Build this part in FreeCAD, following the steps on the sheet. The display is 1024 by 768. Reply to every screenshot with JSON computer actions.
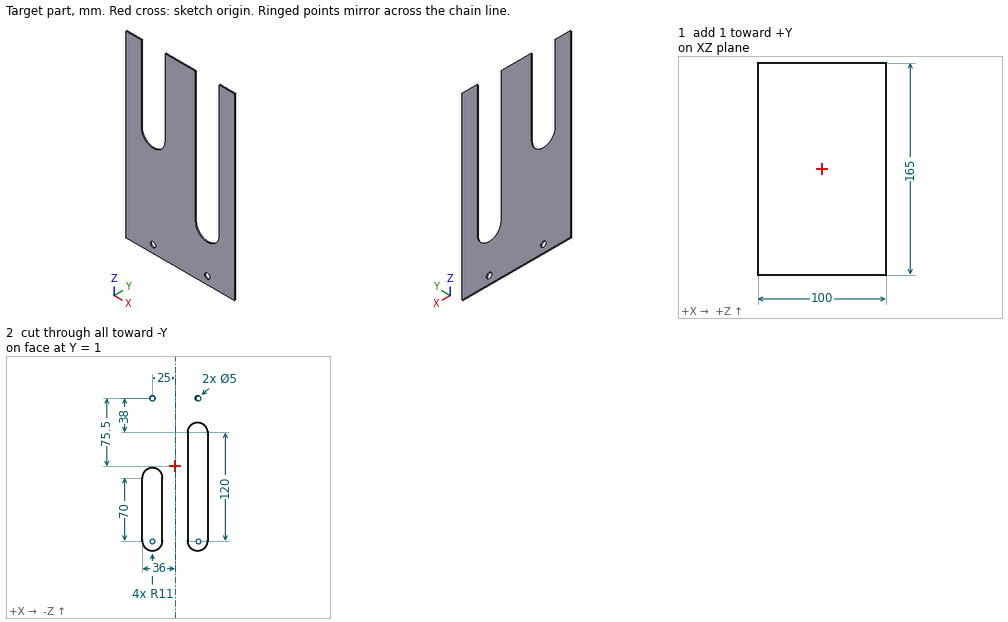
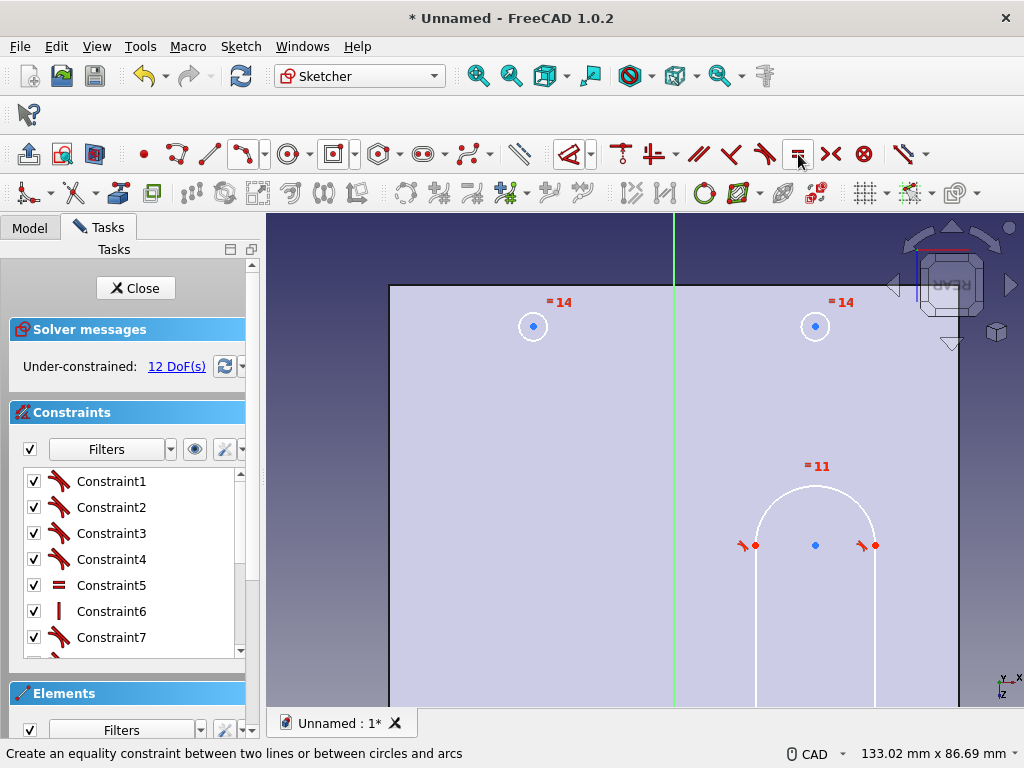
{"action": "scroll", "coordinate": [534, 314], "scroll_direction": "down", "scroll_amount": 6}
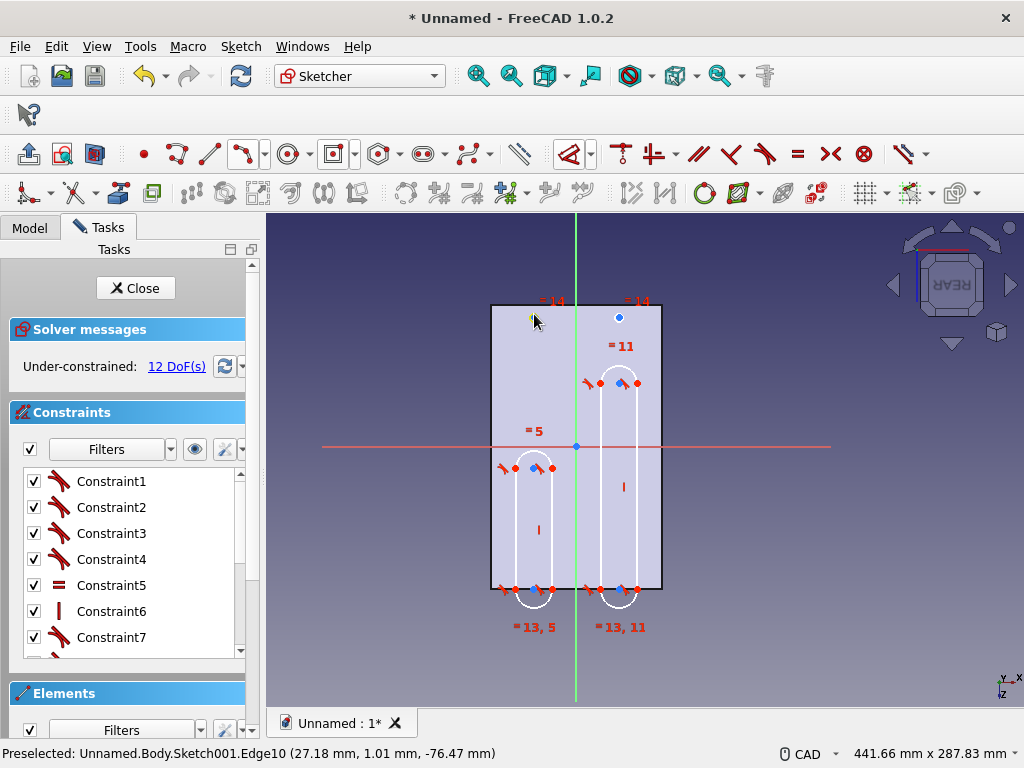
{"action": "left_click", "coordinate": [534, 590]}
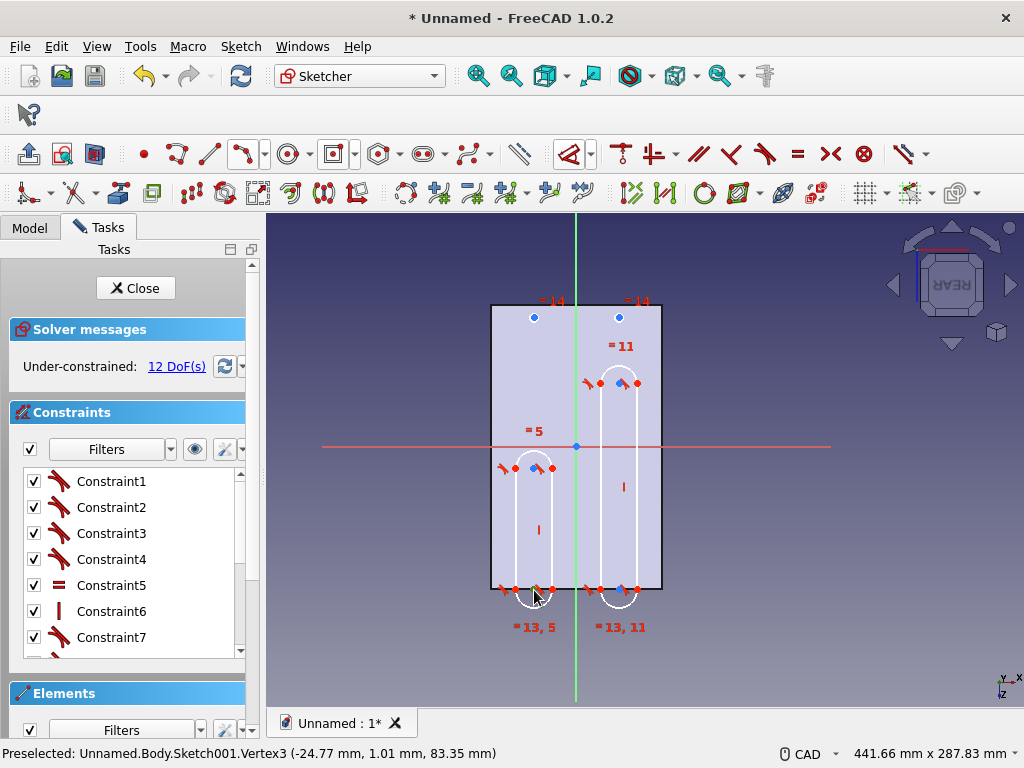
{"action": "left_click", "coordinate": [619, 590]}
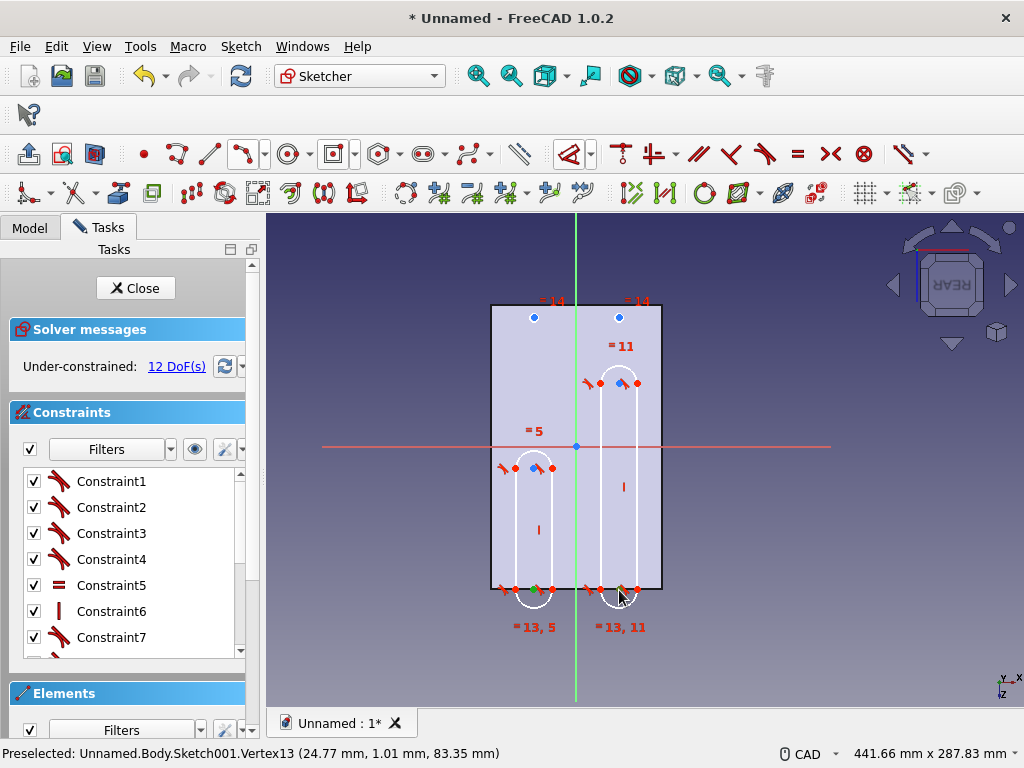
{"action": "left_click", "coordinate": [577, 648]}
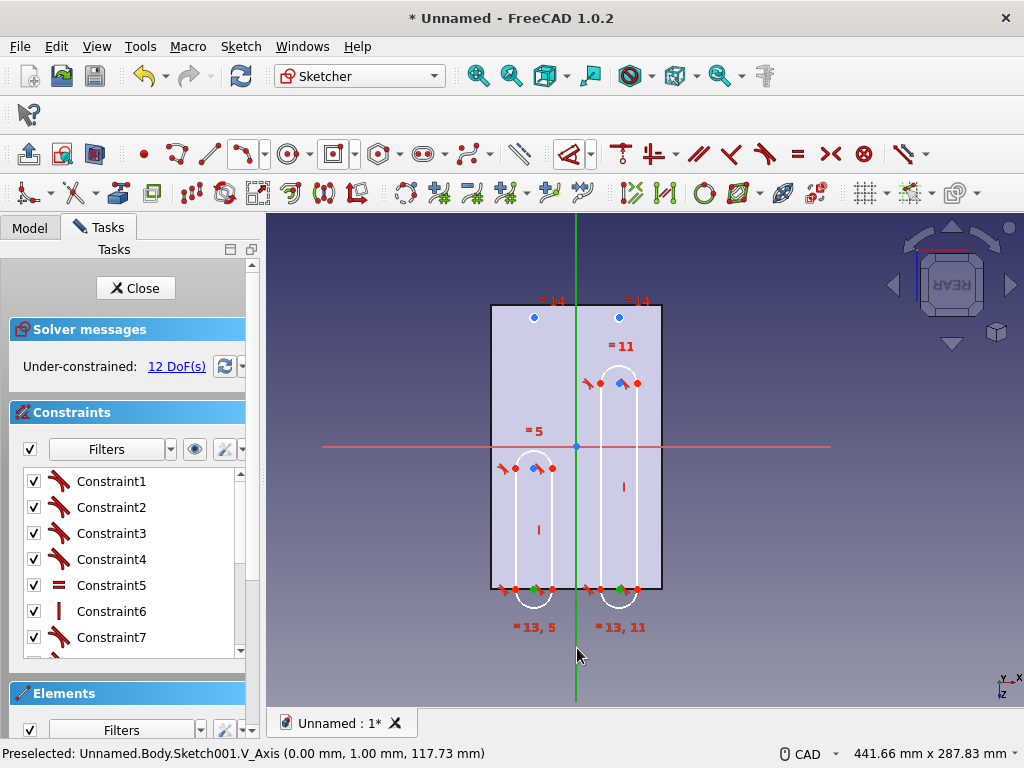
{"action": "left_click", "coordinate": [831, 154]}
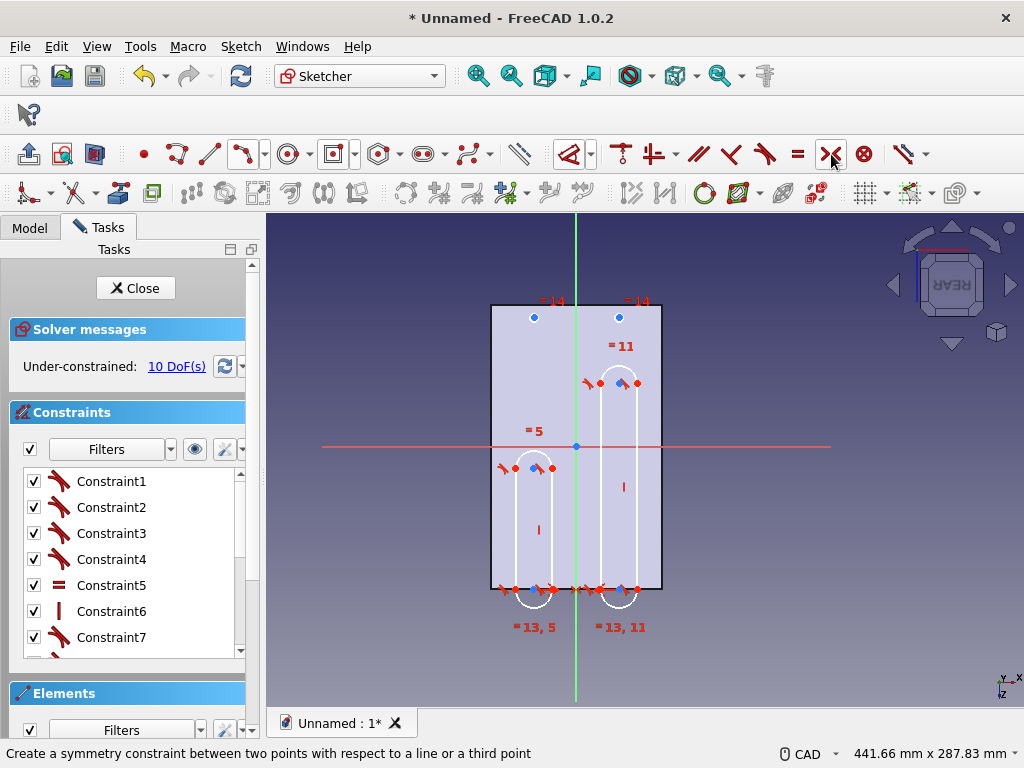
{"action": "left_click", "coordinate": [534, 318]}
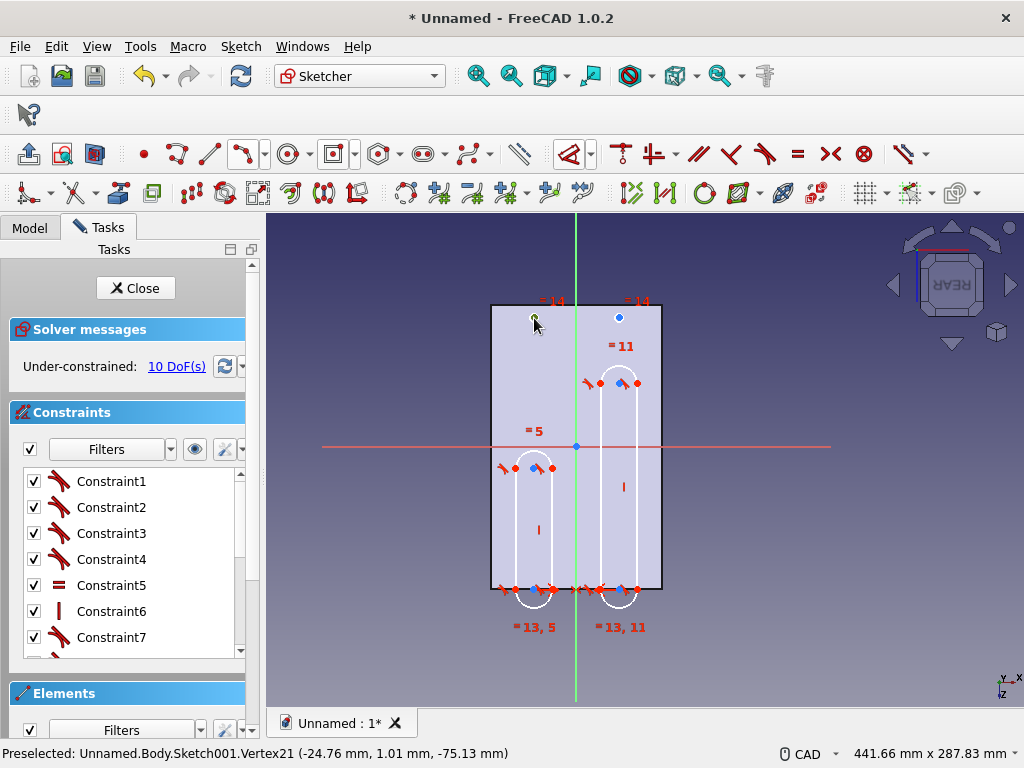
{"action": "left_click", "coordinate": [619, 318]}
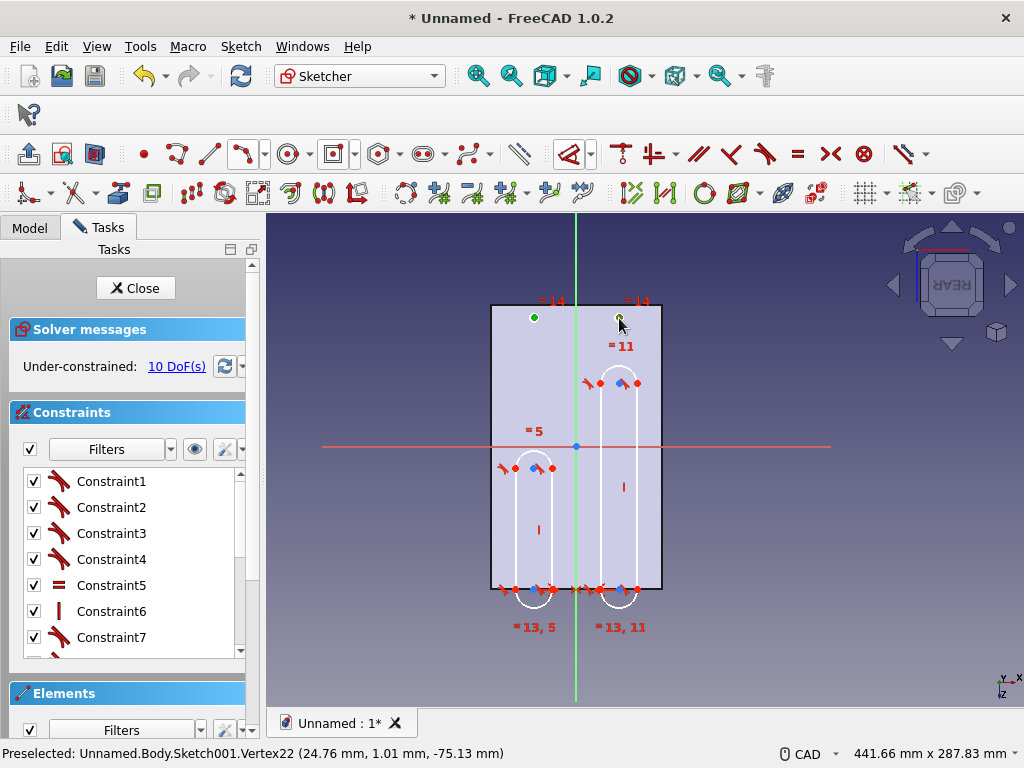
{"action": "left_click", "coordinate": [577, 648]}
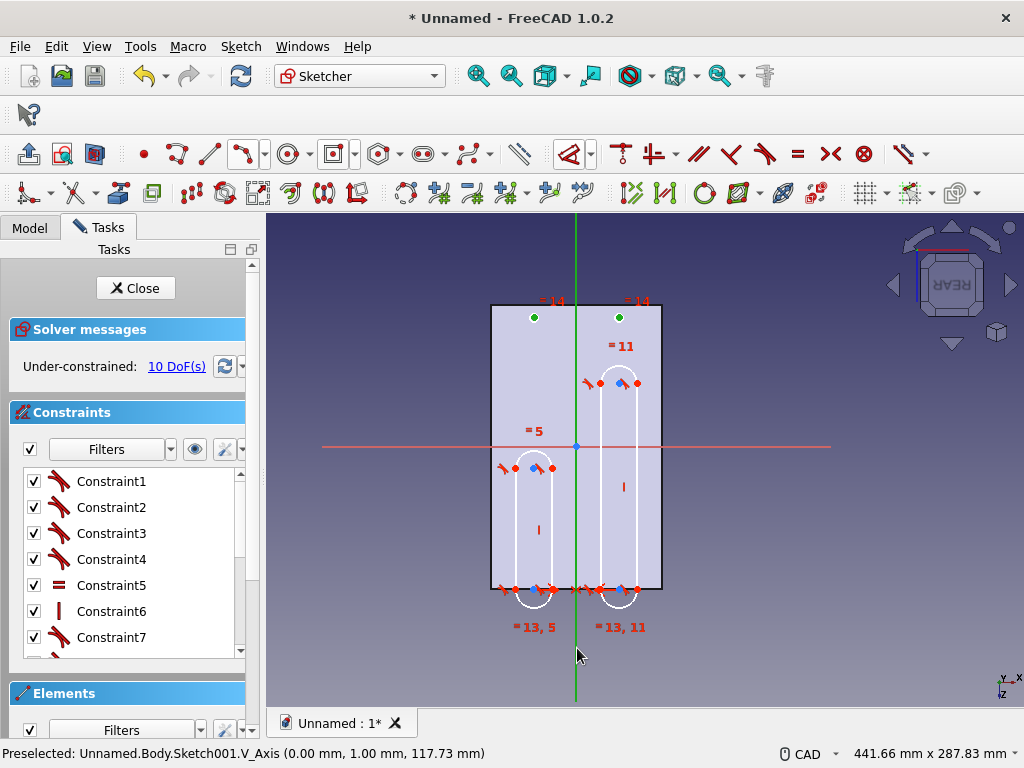
{"action": "left_click", "coordinate": [831, 154]}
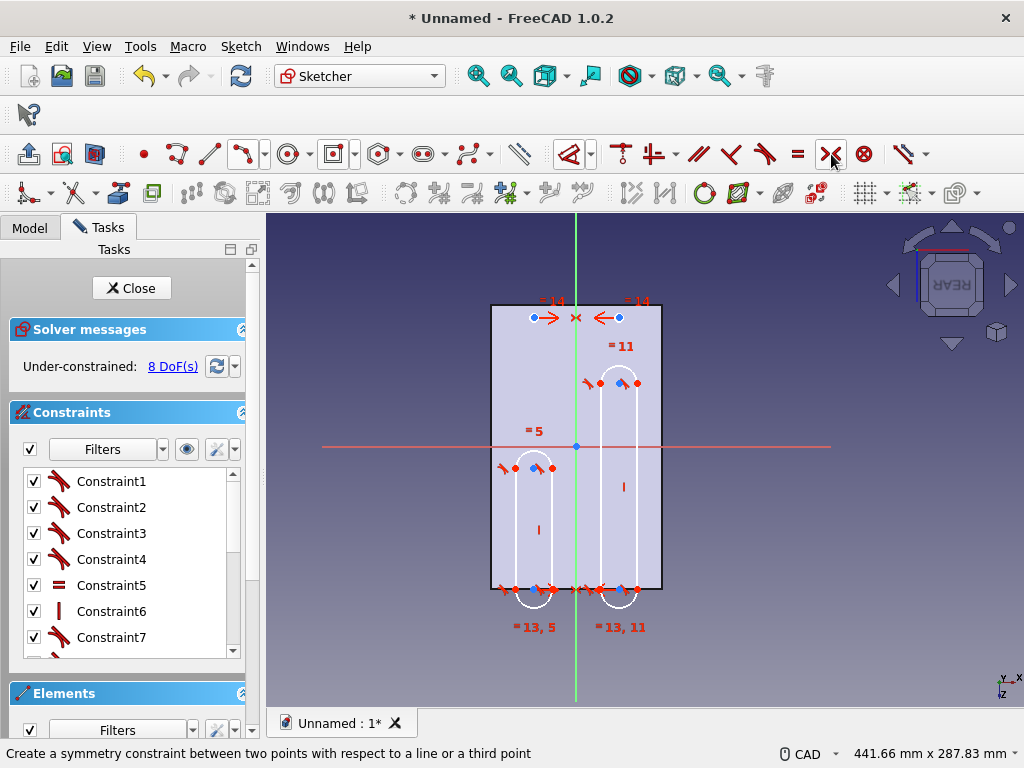
{"action": "scroll", "coordinate": [523, 605], "scroll_direction": "up", "scroll_amount": 4}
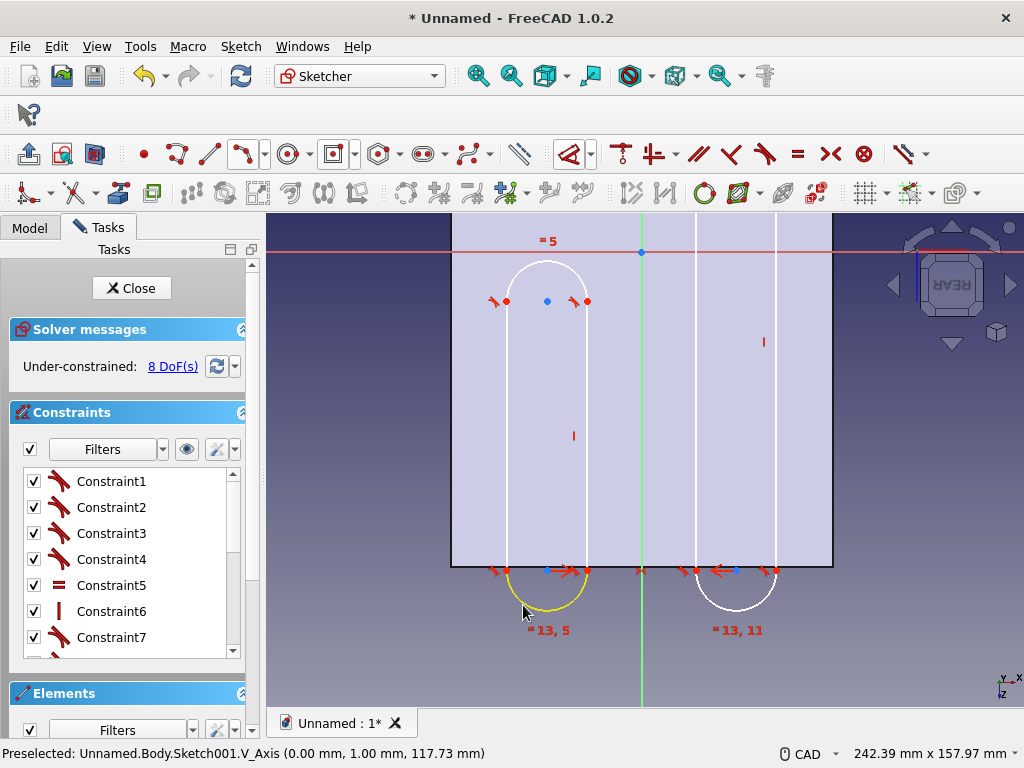
{"action": "left_click", "coordinate": [523, 603]}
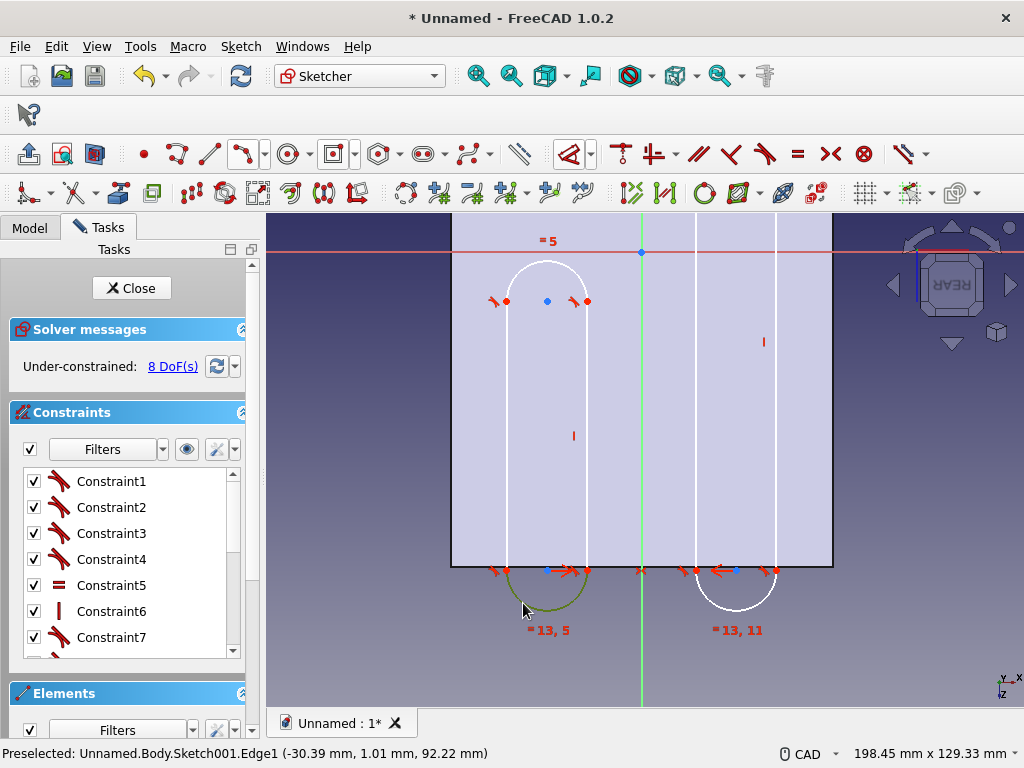
{"action": "left_click", "coordinate": [590, 154]}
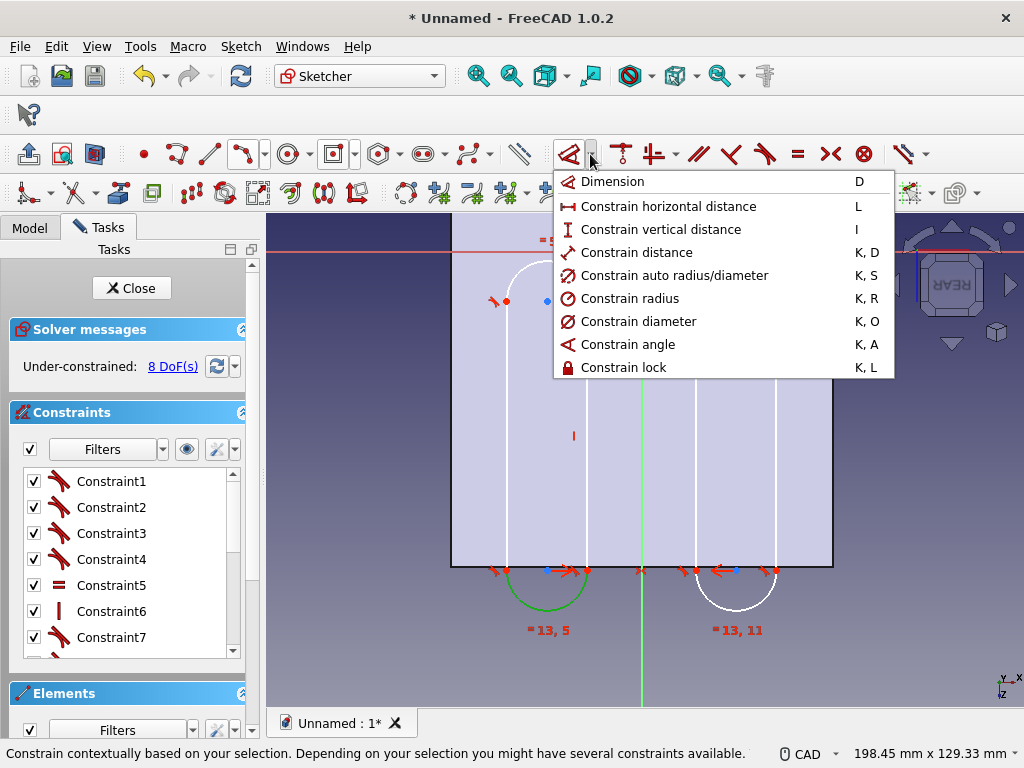
{"action": "left_click", "coordinate": [724, 298]}